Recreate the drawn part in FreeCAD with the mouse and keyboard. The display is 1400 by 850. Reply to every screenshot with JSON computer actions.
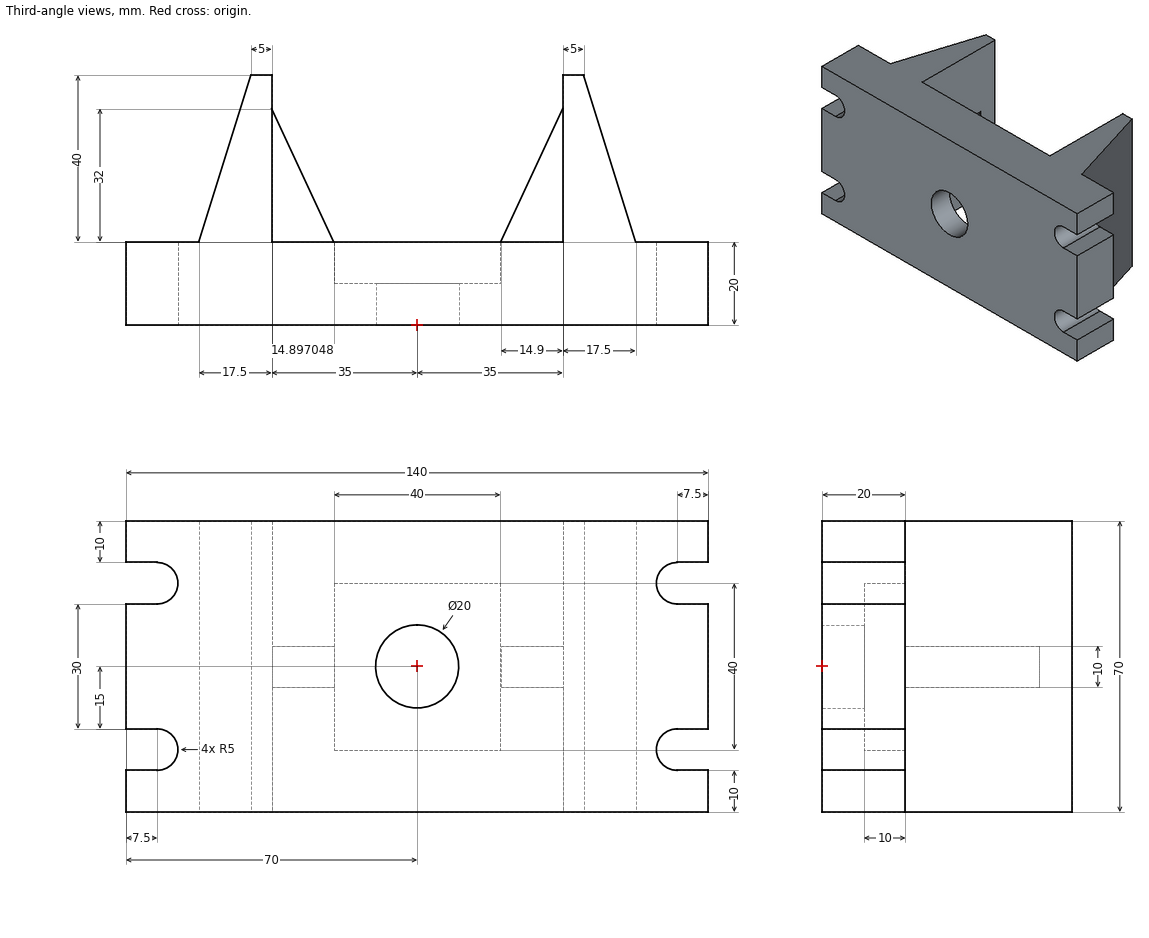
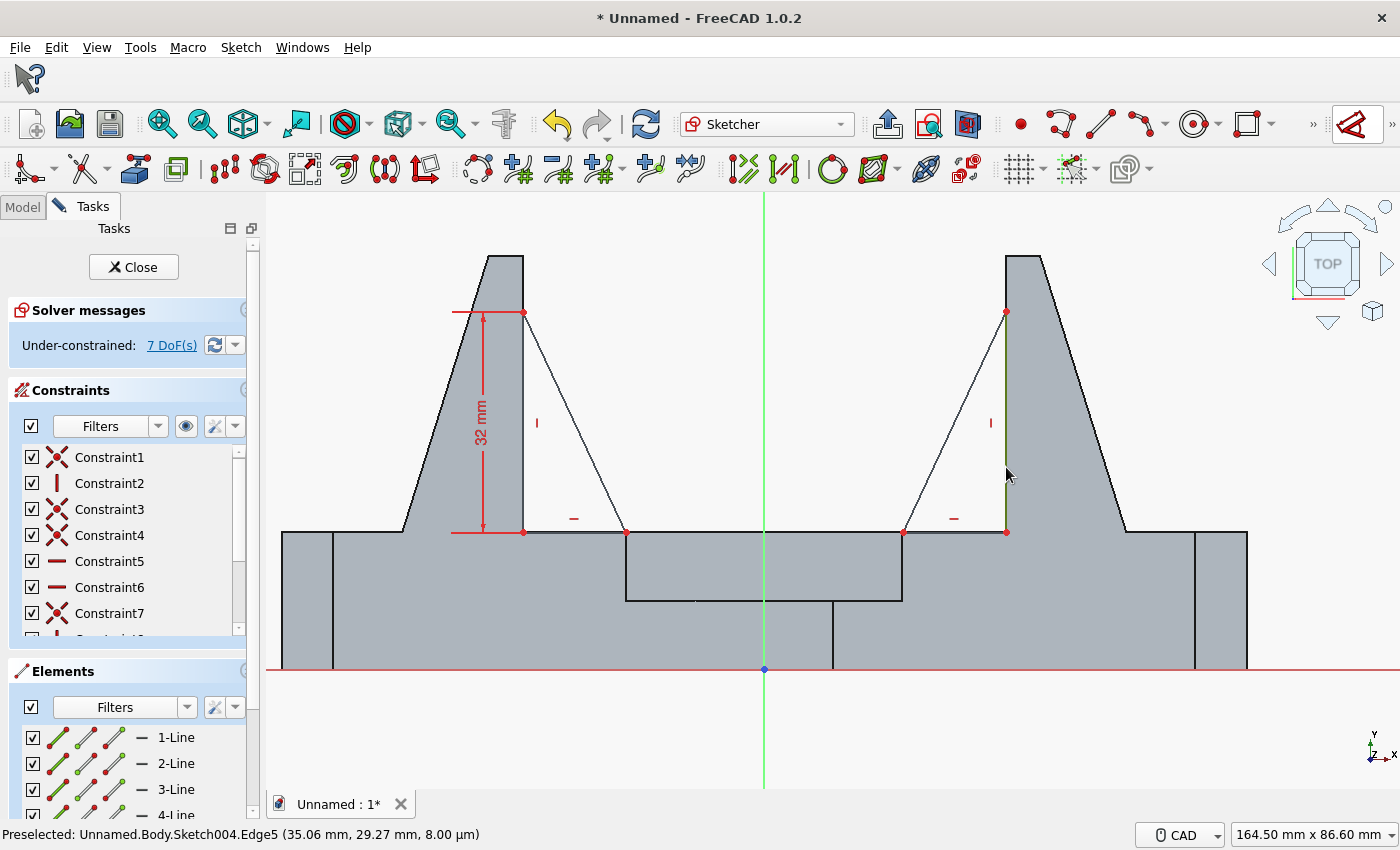
{"action": "key", "text": "i"}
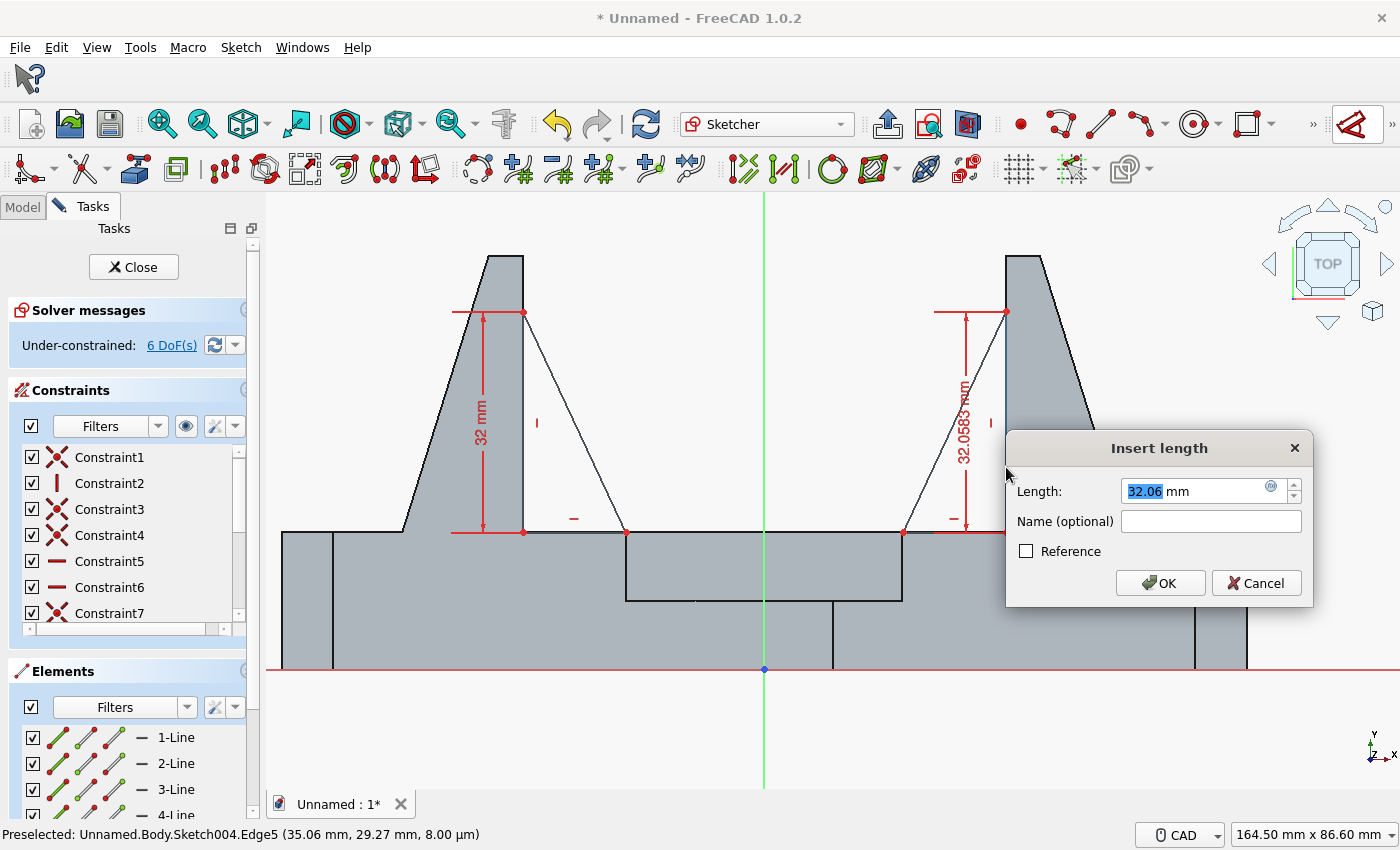
{"action": "type", "text": "32"}
{"action": "key", "text": "Return"}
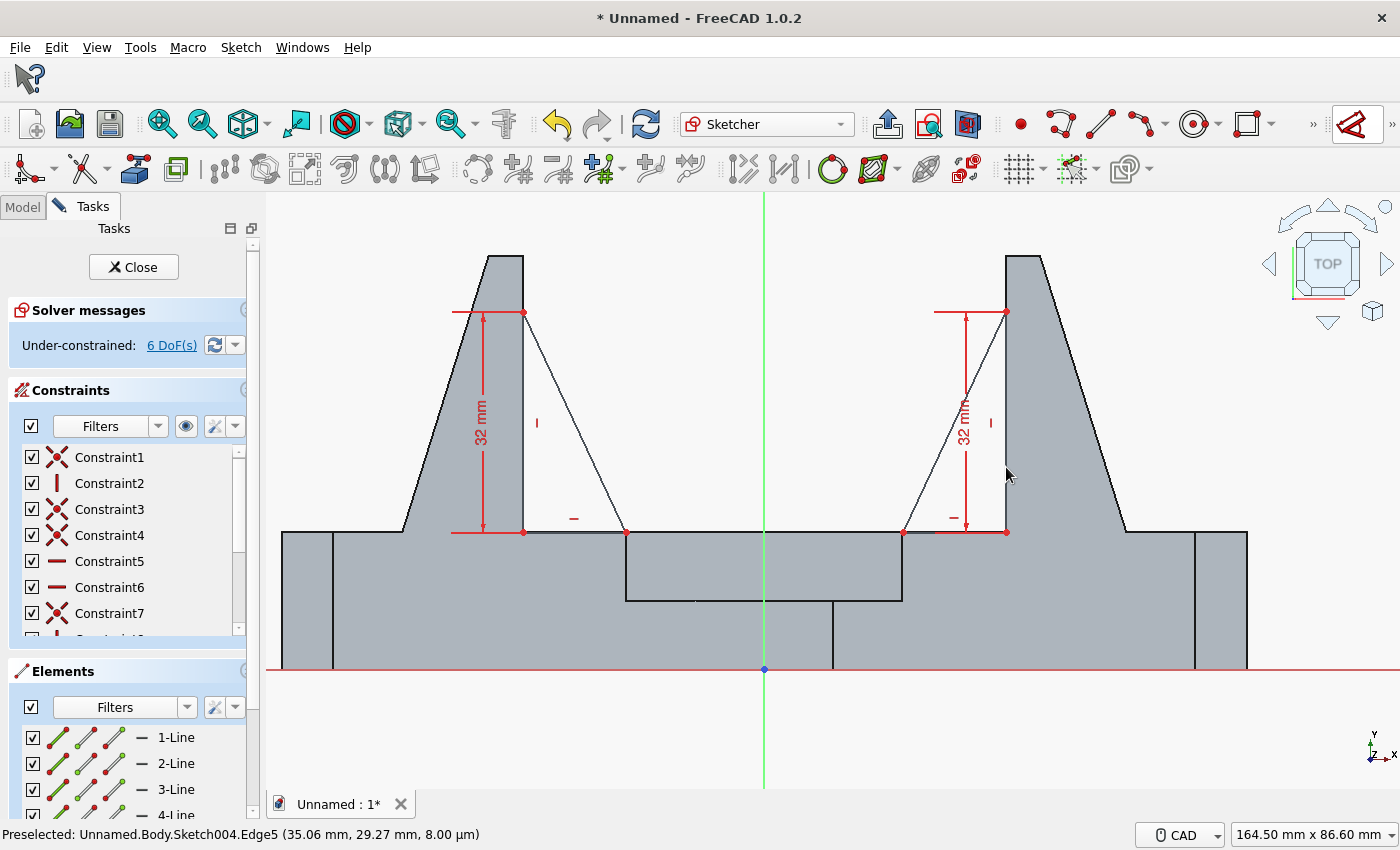
{"action": "left_click", "coordinate": [626, 533]}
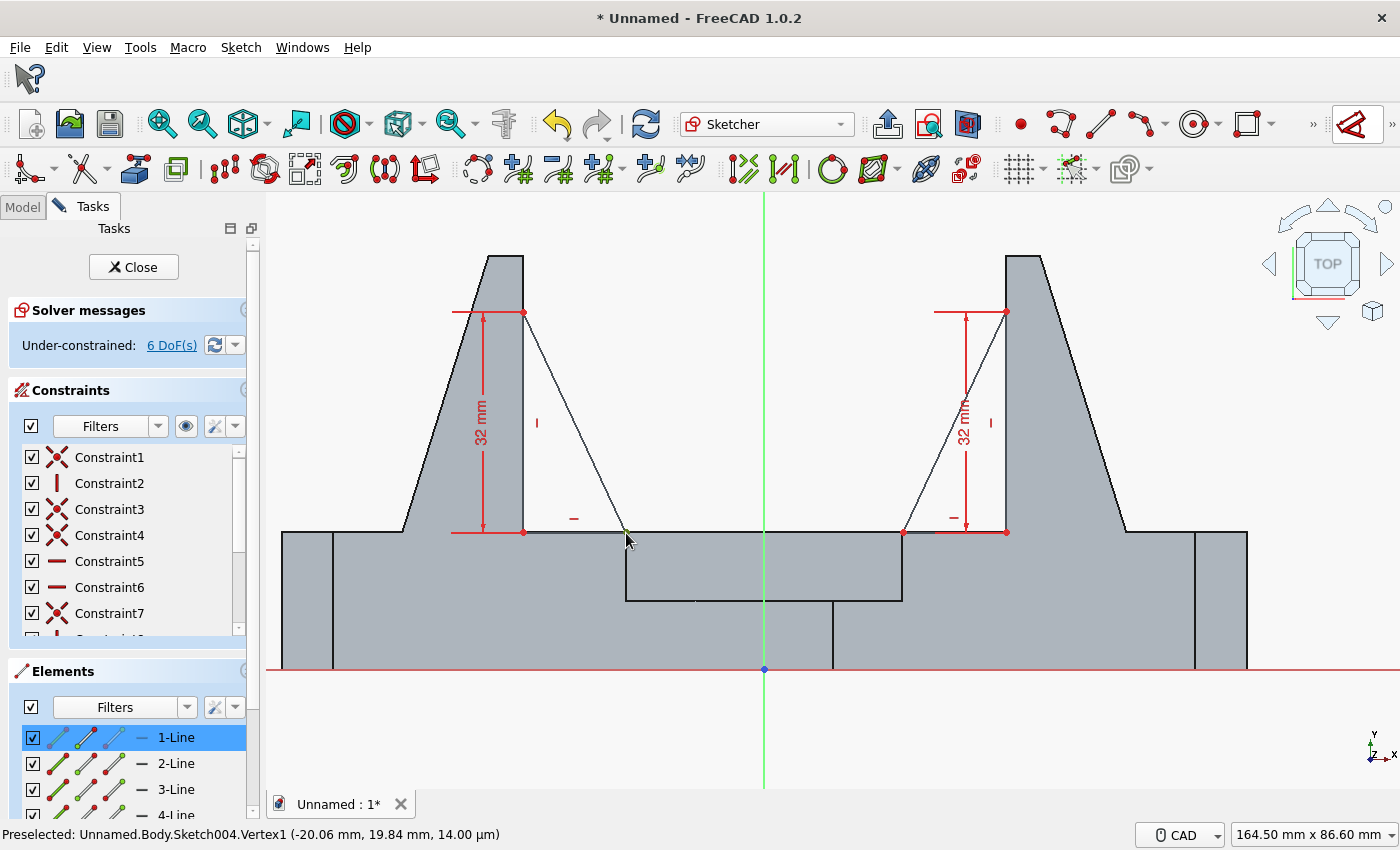
{"action": "left_click", "coordinate": [1378, 124]}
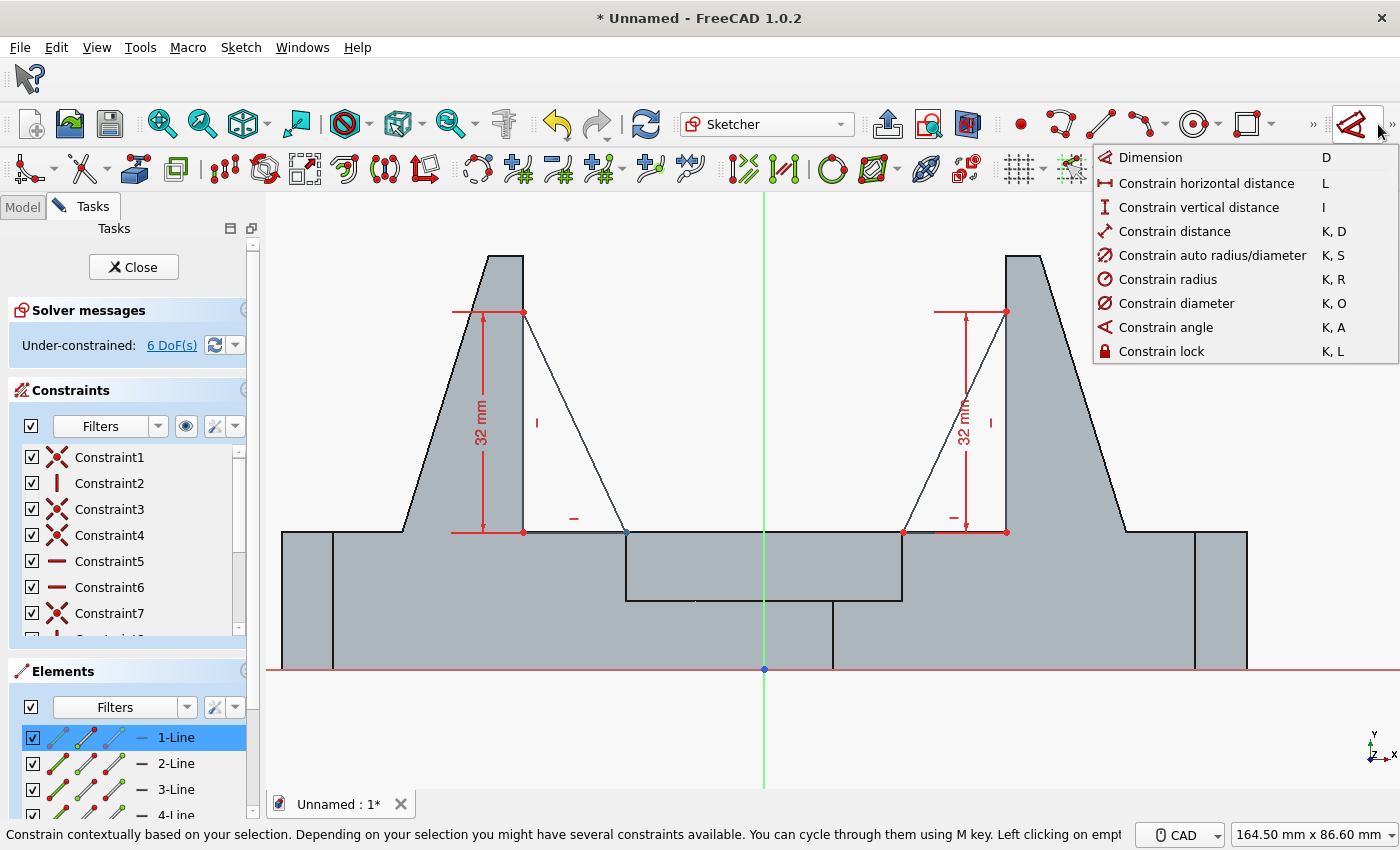
{"action": "left_click", "coordinate": [1246, 207]}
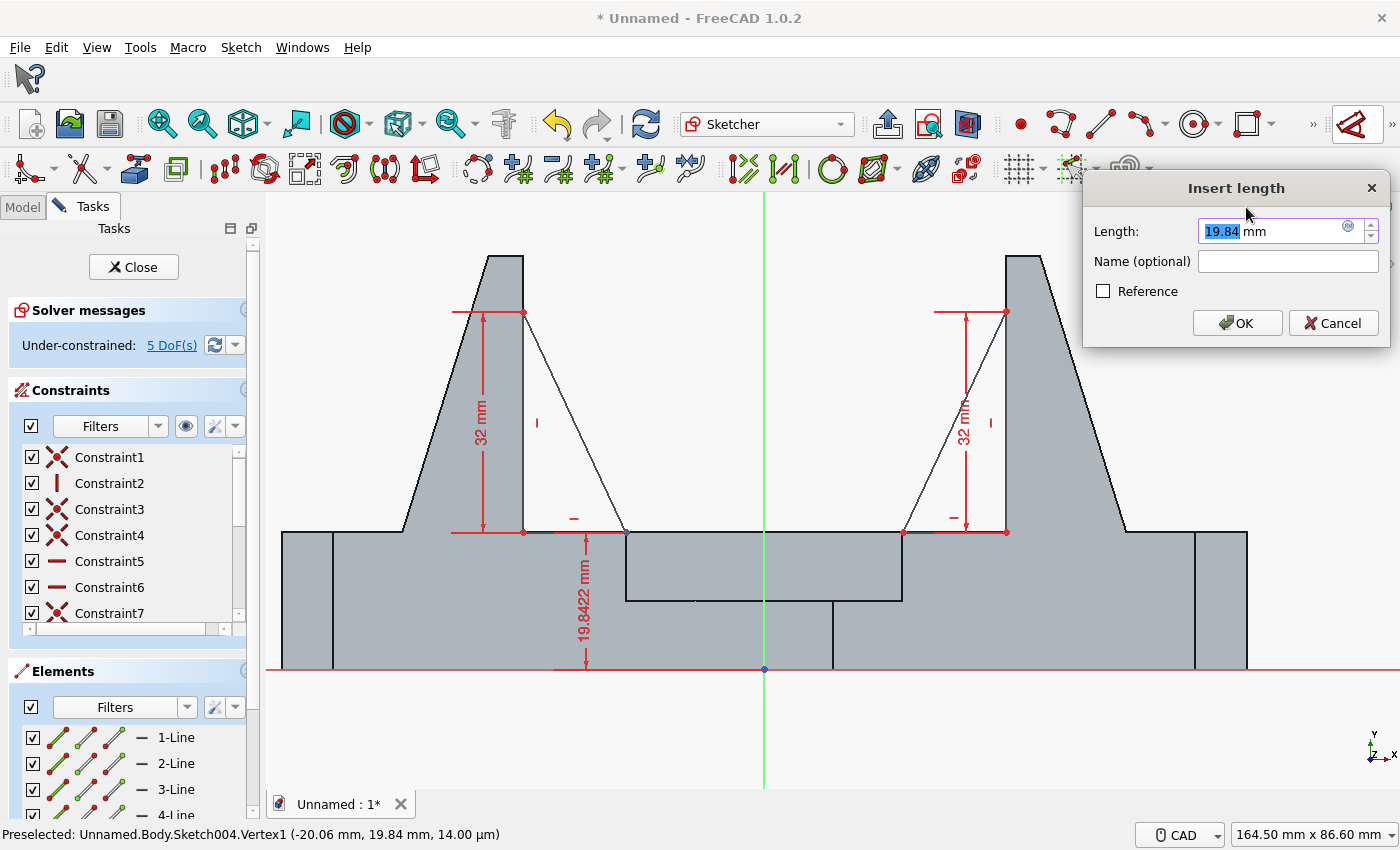
{"action": "type", "text": "20"}
{"action": "key", "text": "Return"}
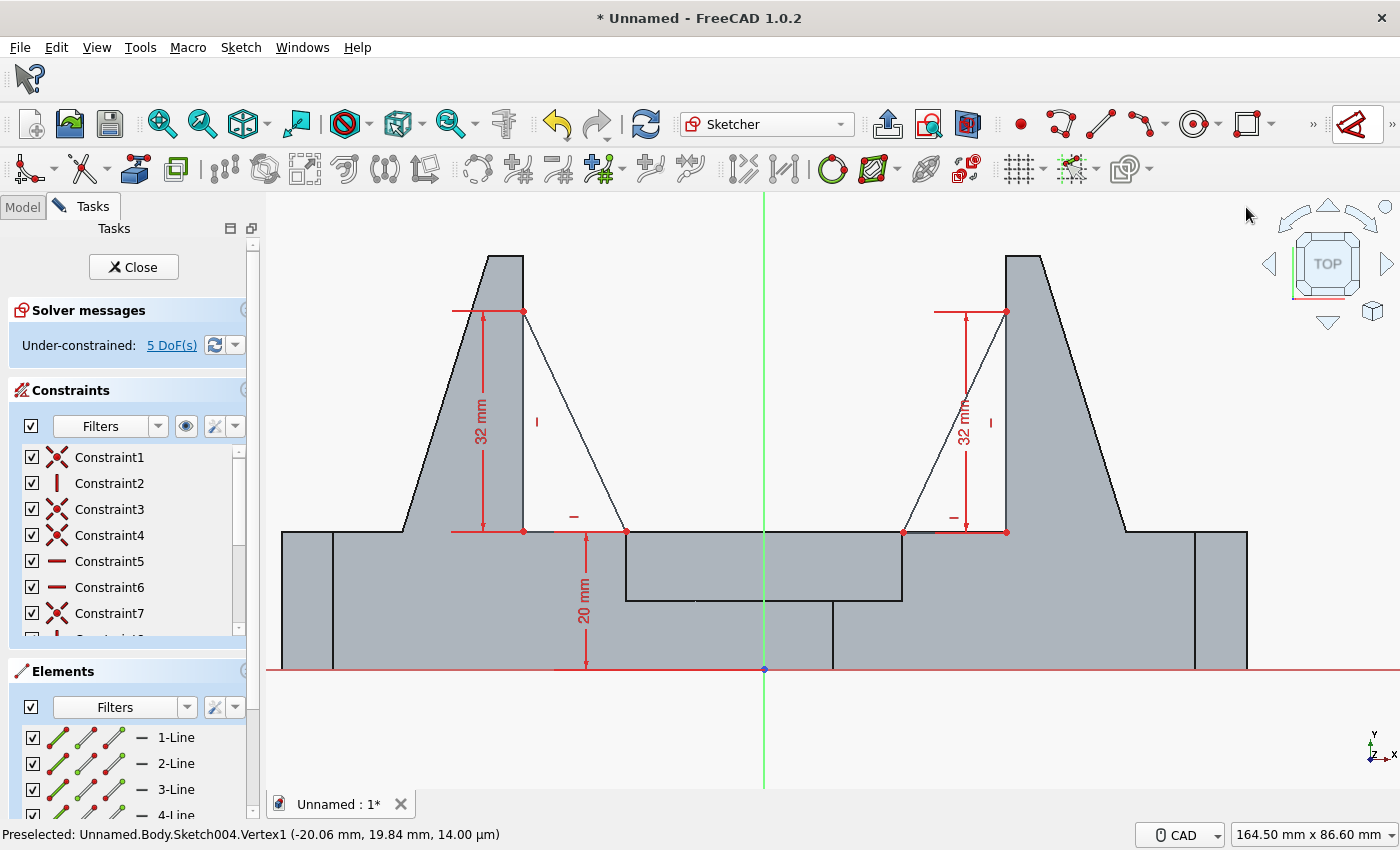
{"action": "left_click", "coordinate": [523, 311]}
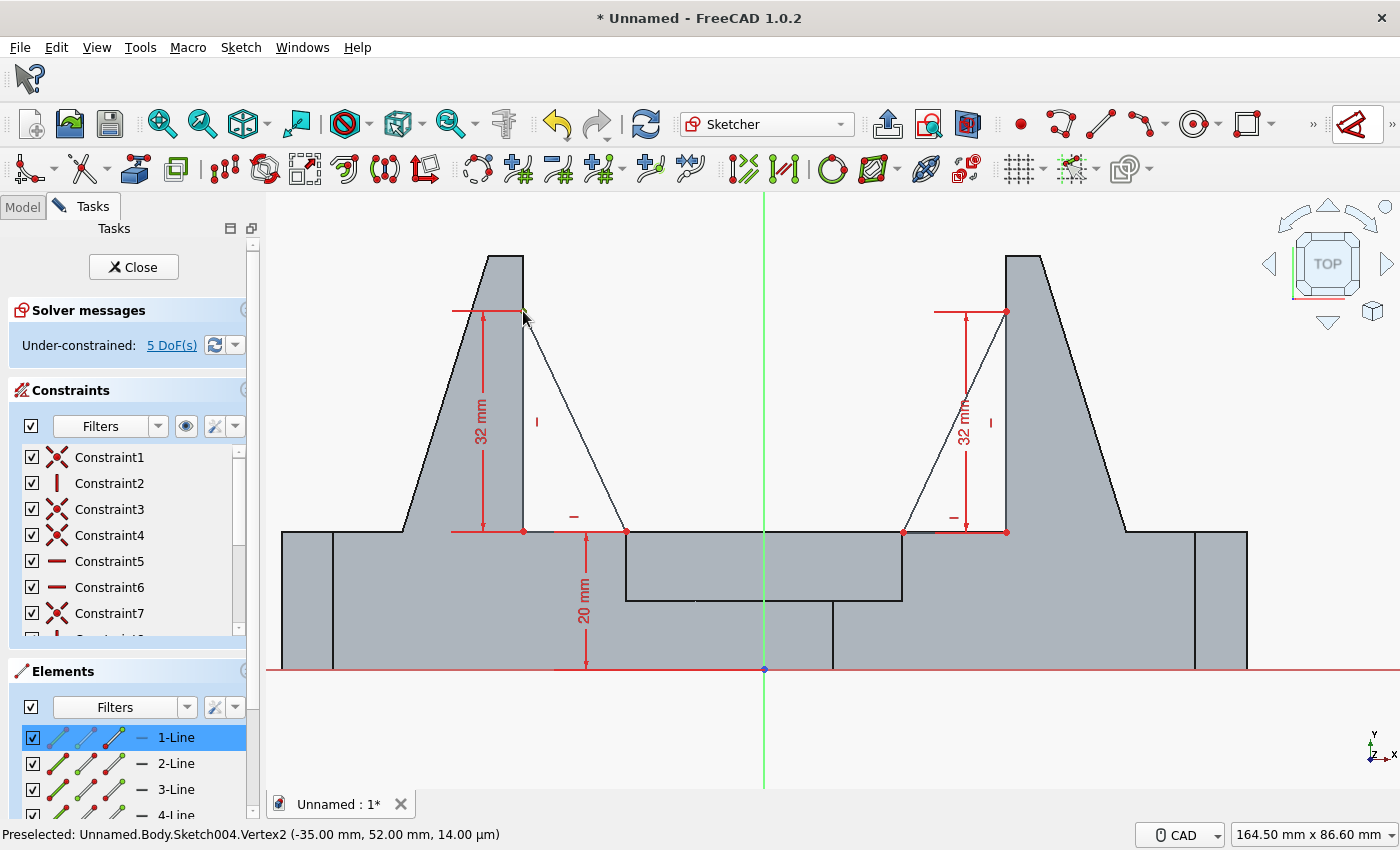
{"action": "key", "text": "l"}